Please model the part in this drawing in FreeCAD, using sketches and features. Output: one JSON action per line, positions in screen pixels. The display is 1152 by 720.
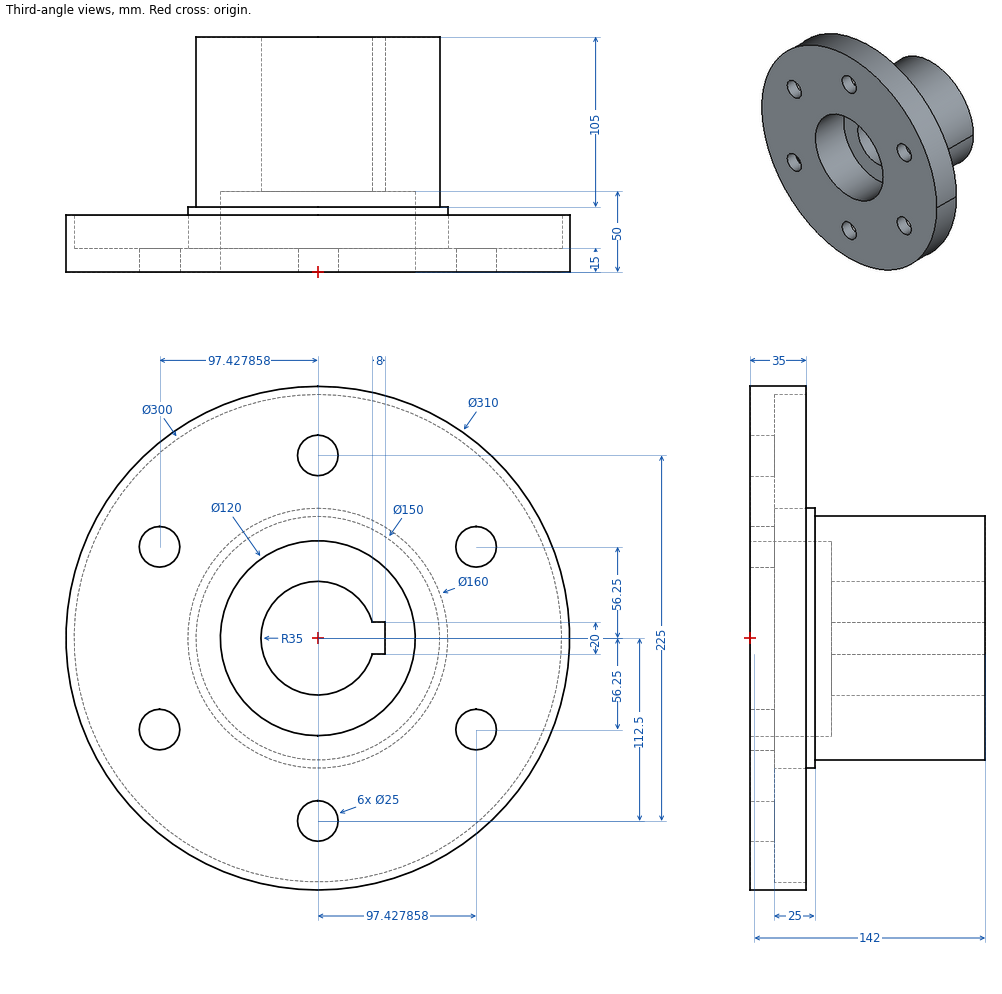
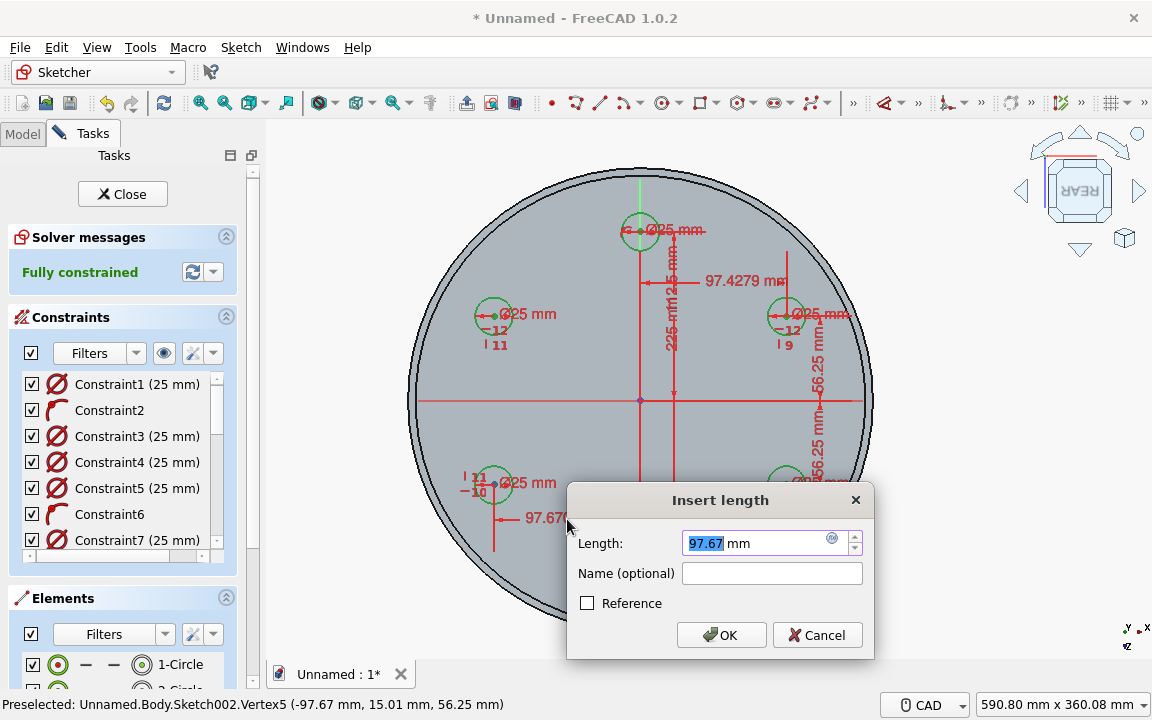
{"action": "type", "text": "97.427858"}
{"action": "key", "text": "Return"}
{"action": "key", "text": "Escape"}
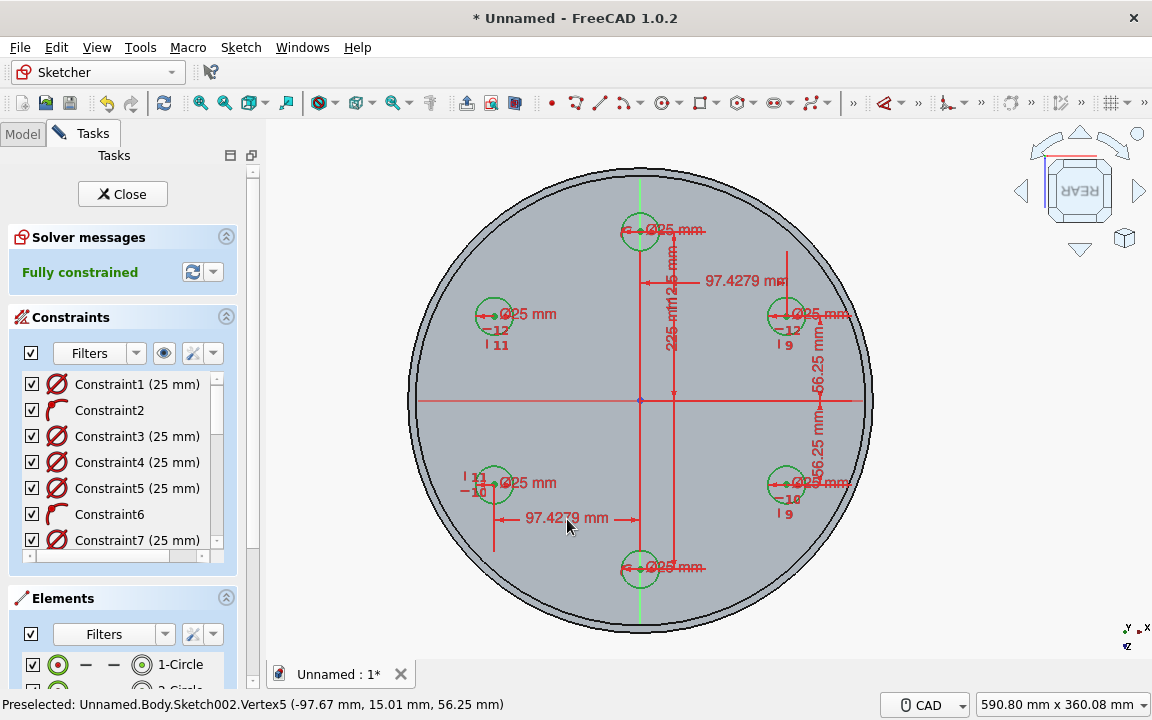
{"action": "left_click", "coordinate": [123, 194]}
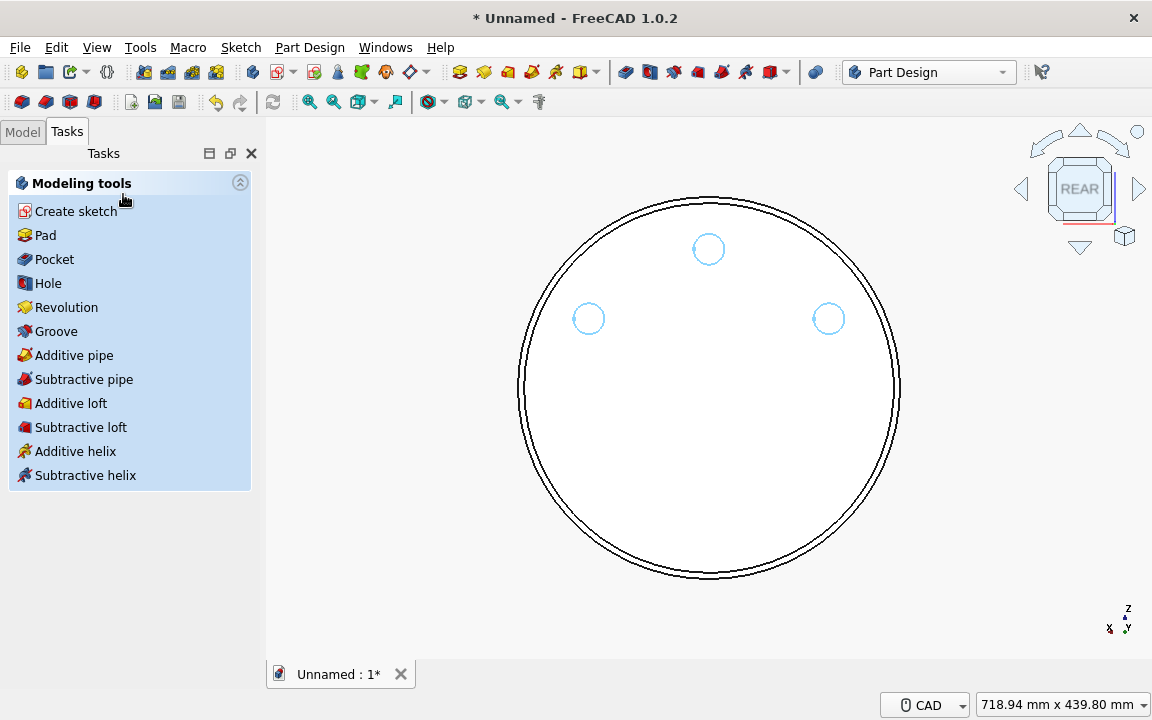
{"action": "left_click", "coordinate": [626, 72]}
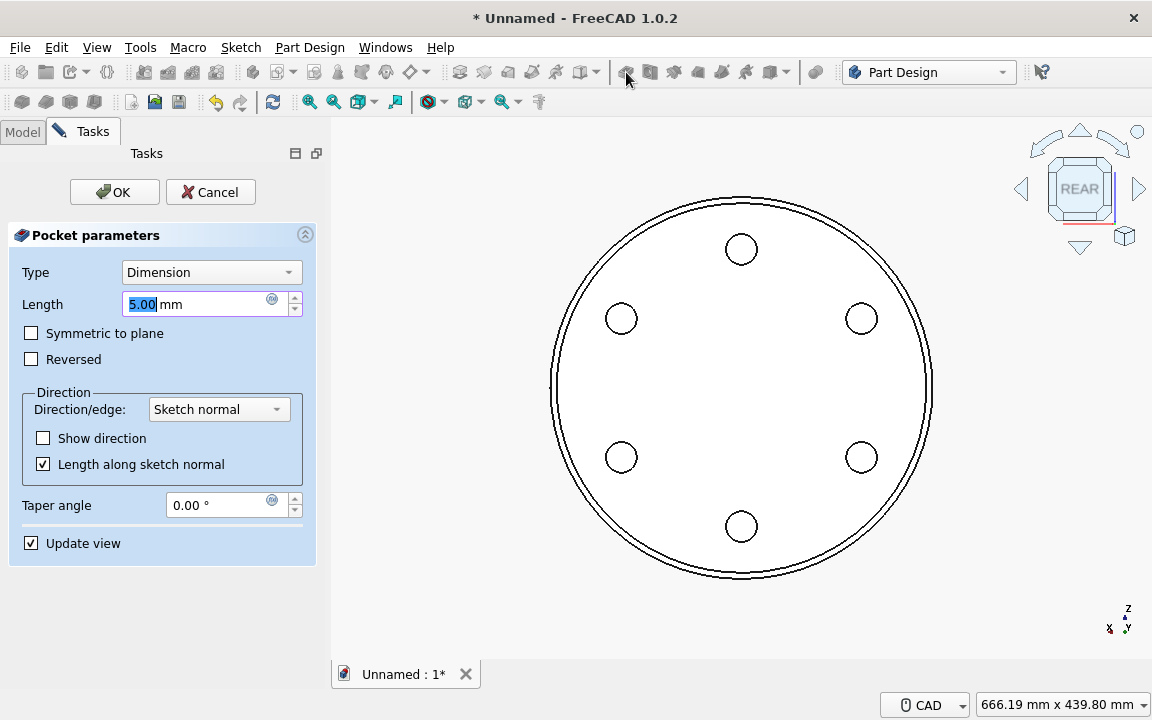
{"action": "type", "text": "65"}
{"action": "key", "text": "Tab"}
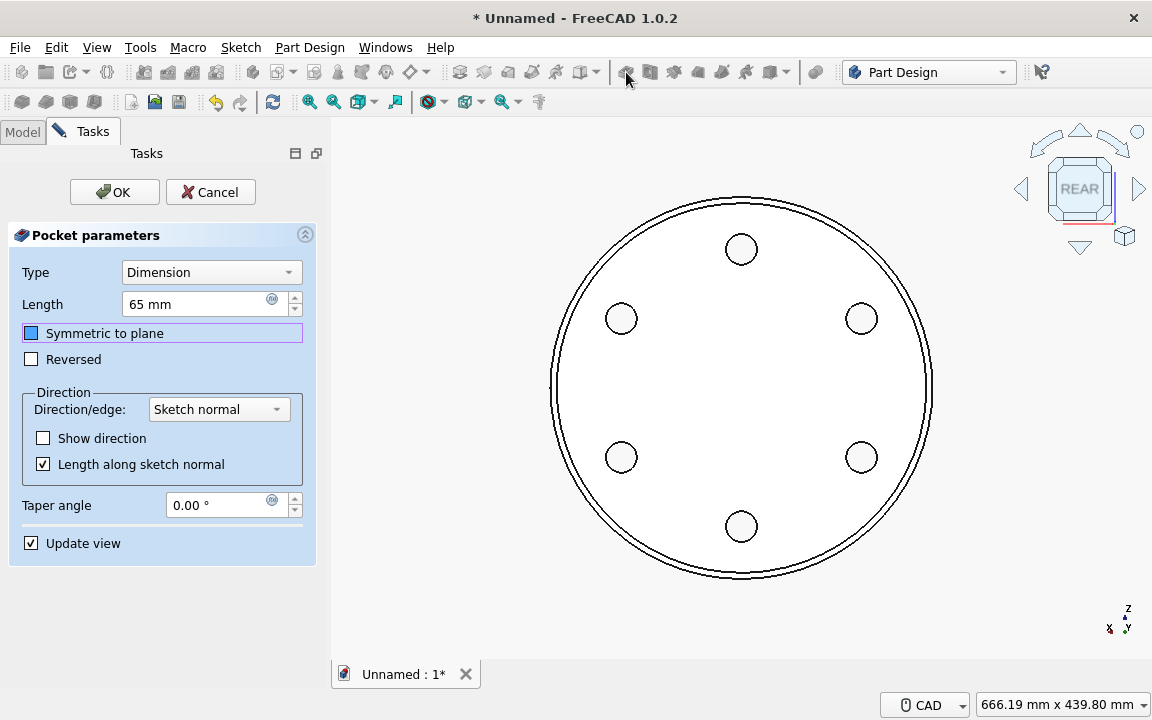
{"action": "left_click", "coordinate": [115, 192]}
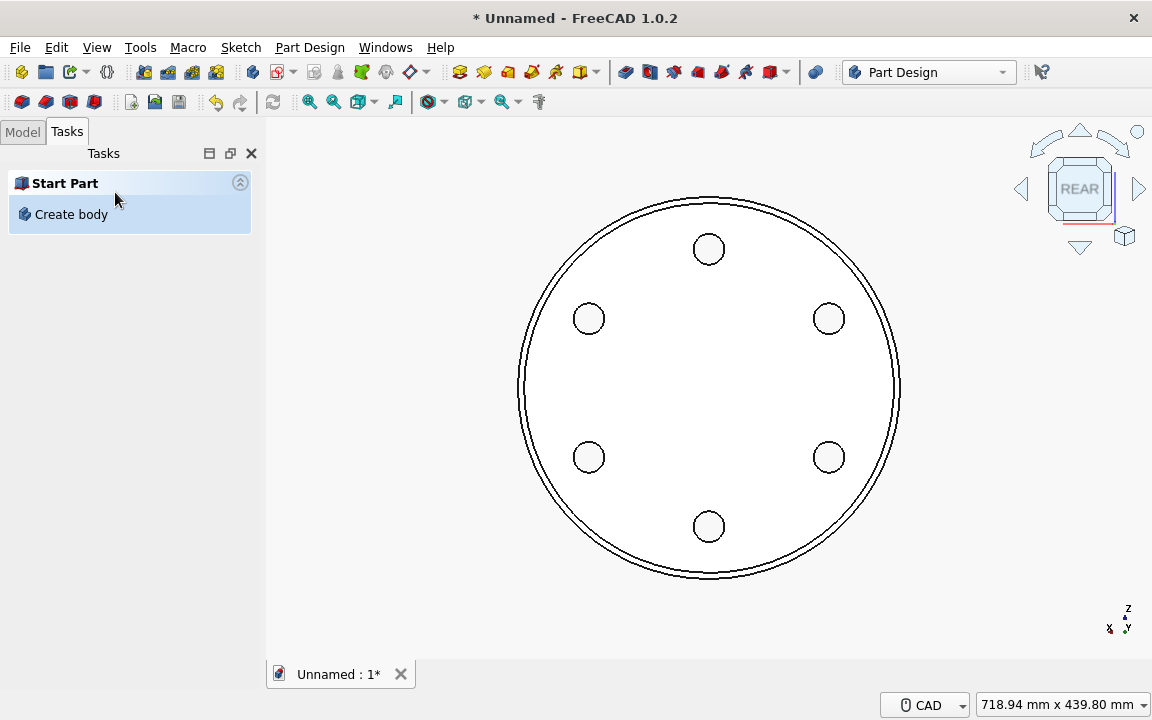
{"action": "left_click", "coordinate": [709, 387]}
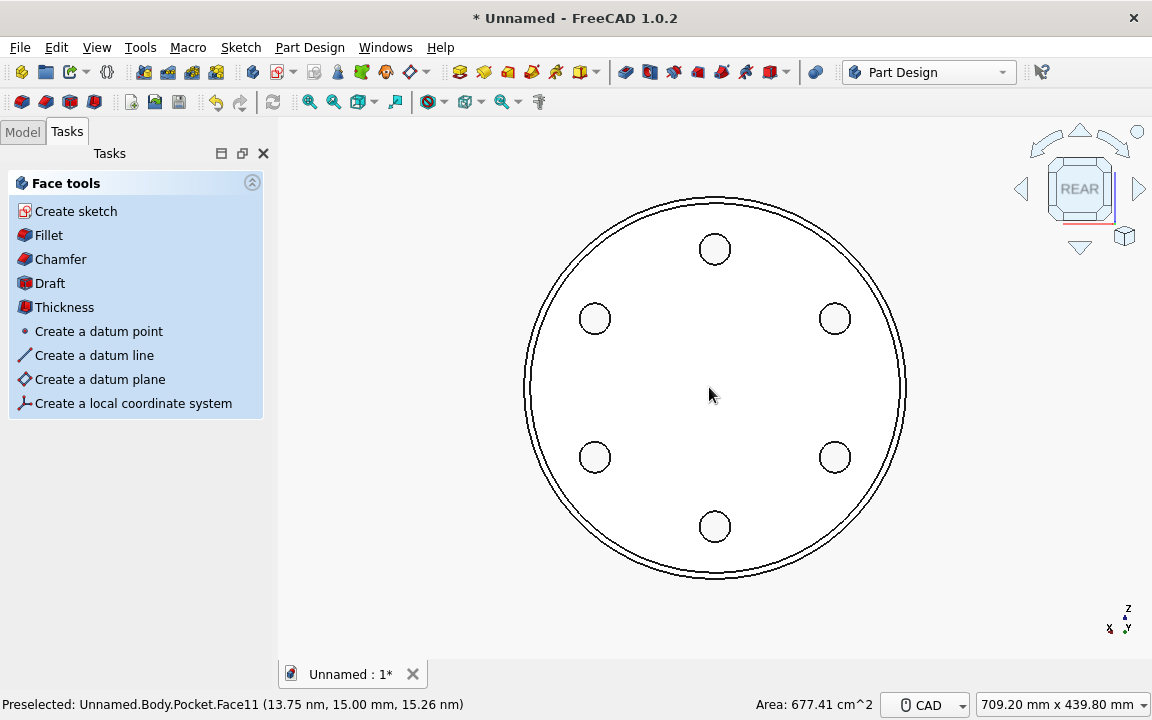
{"action": "left_click", "coordinate": [278, 72]}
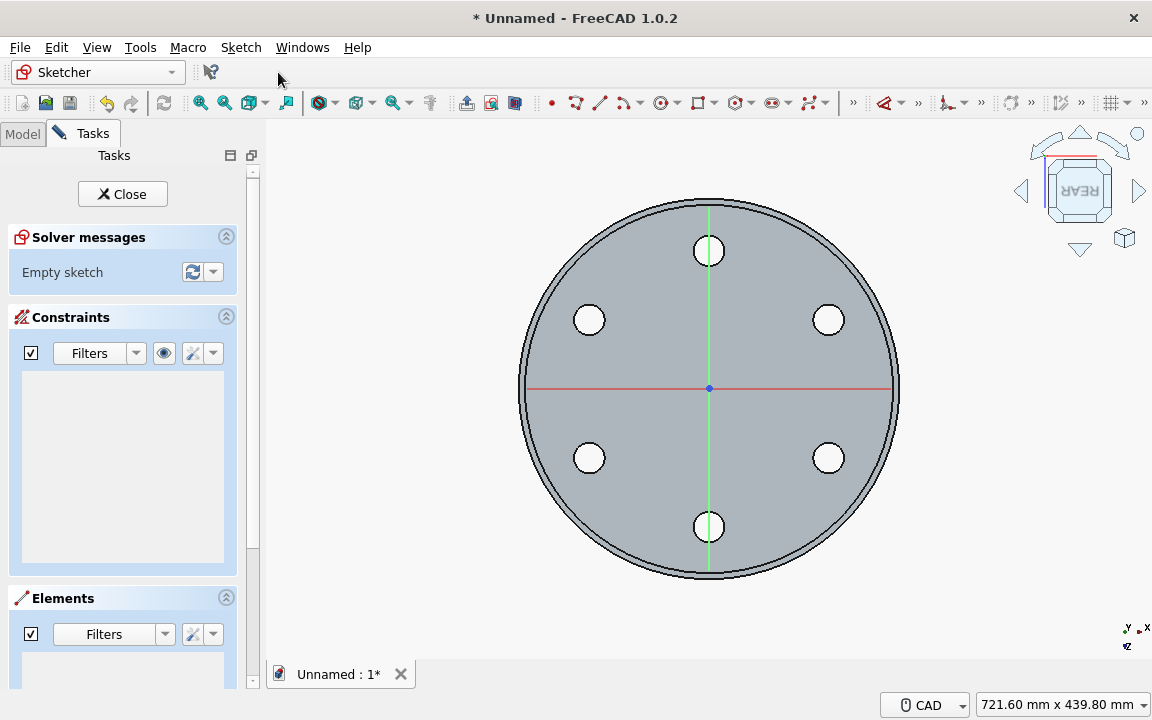
{"action": "scroll", "coordinate": [792, 389], "scroll_direction": "up", "scroll_amount": 3}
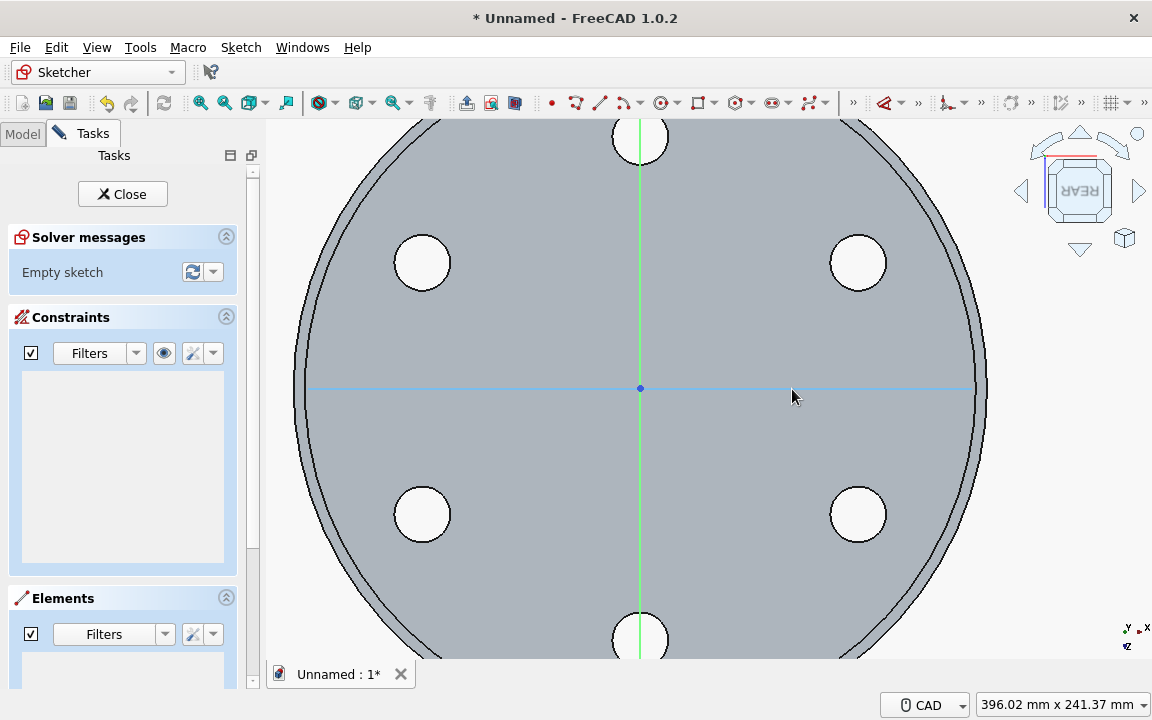
{"action": "left_click", "coordinate": [662, 104]}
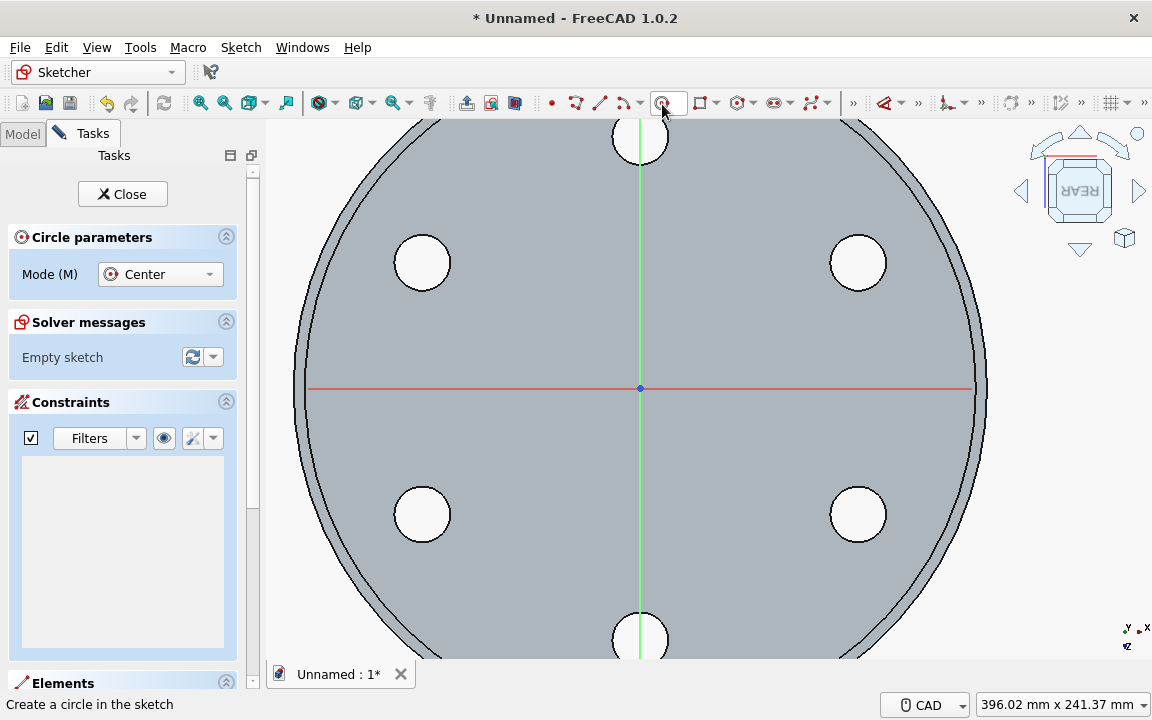
{"action": "left_click", "coordinate": [640, 389]}
{"action": "mouse_move", "coordinate": [767, 262]}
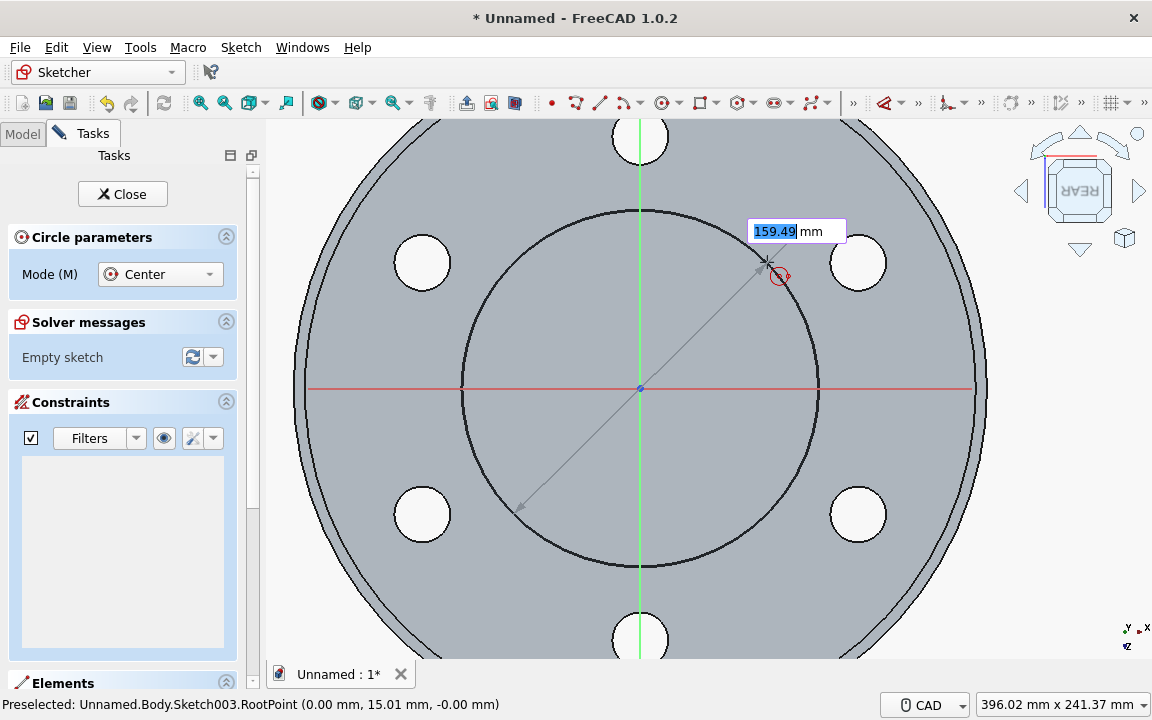
{"action": "type", "text": "160"}
{"action": "key", "text": "Return"}
{"action": "key", "text": "Escape"}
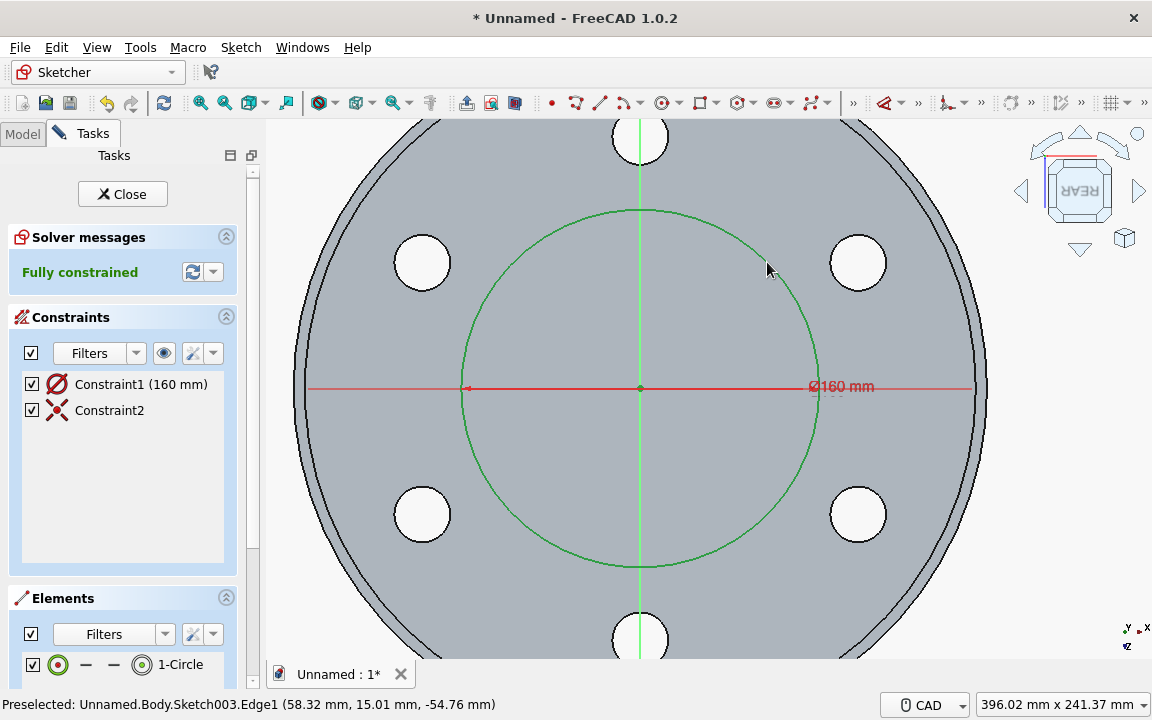
{"action": "left_click", "coordinate": [123, 194]}